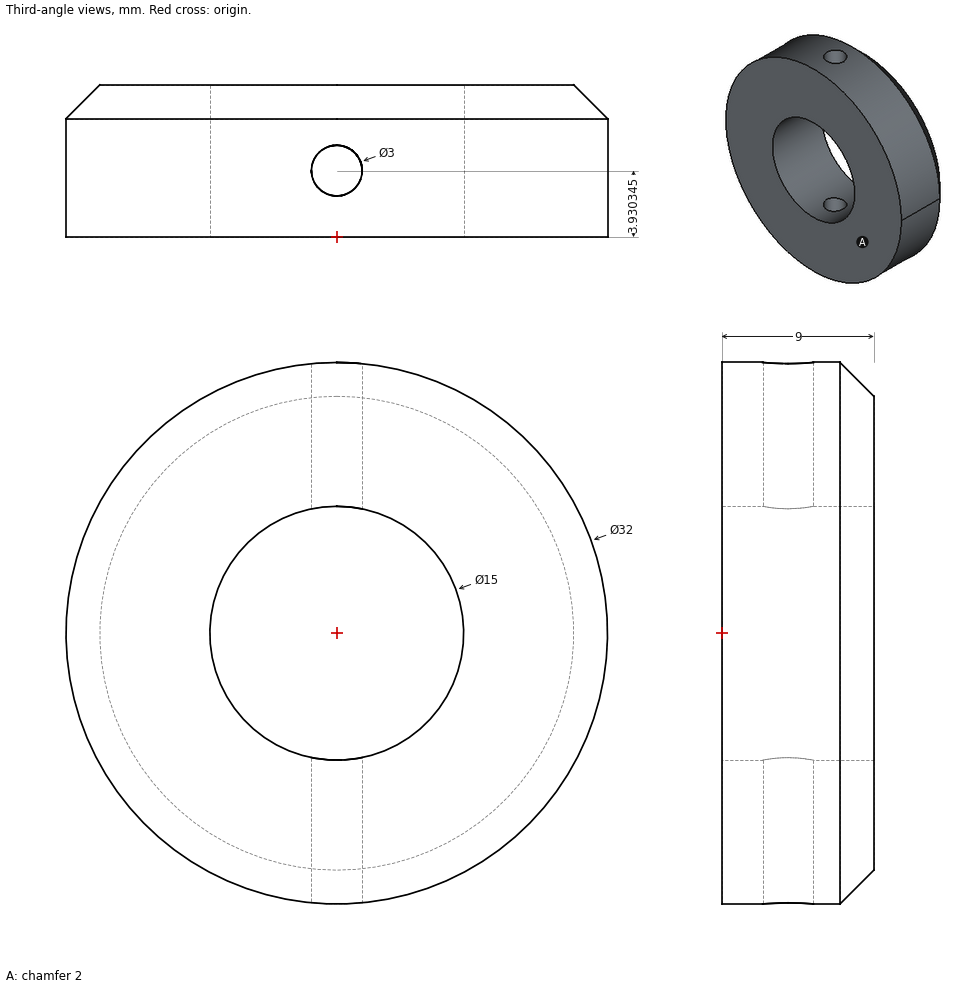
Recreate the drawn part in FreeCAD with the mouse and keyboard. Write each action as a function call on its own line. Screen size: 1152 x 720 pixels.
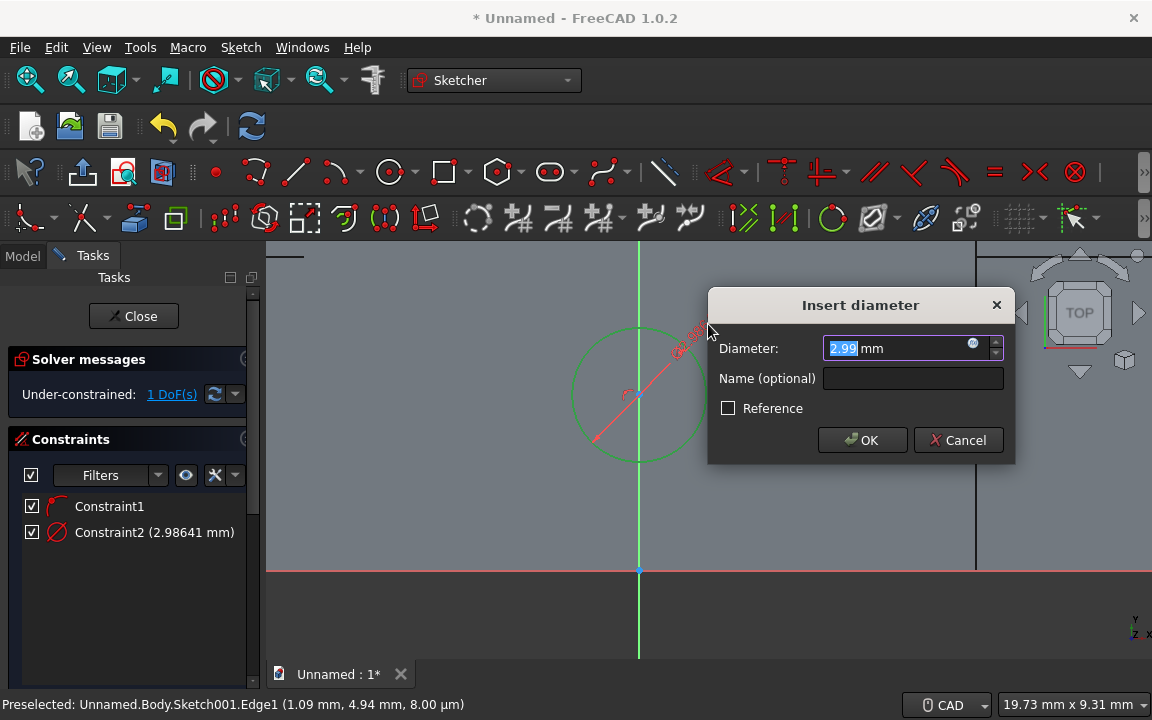
text(3)
key(Return)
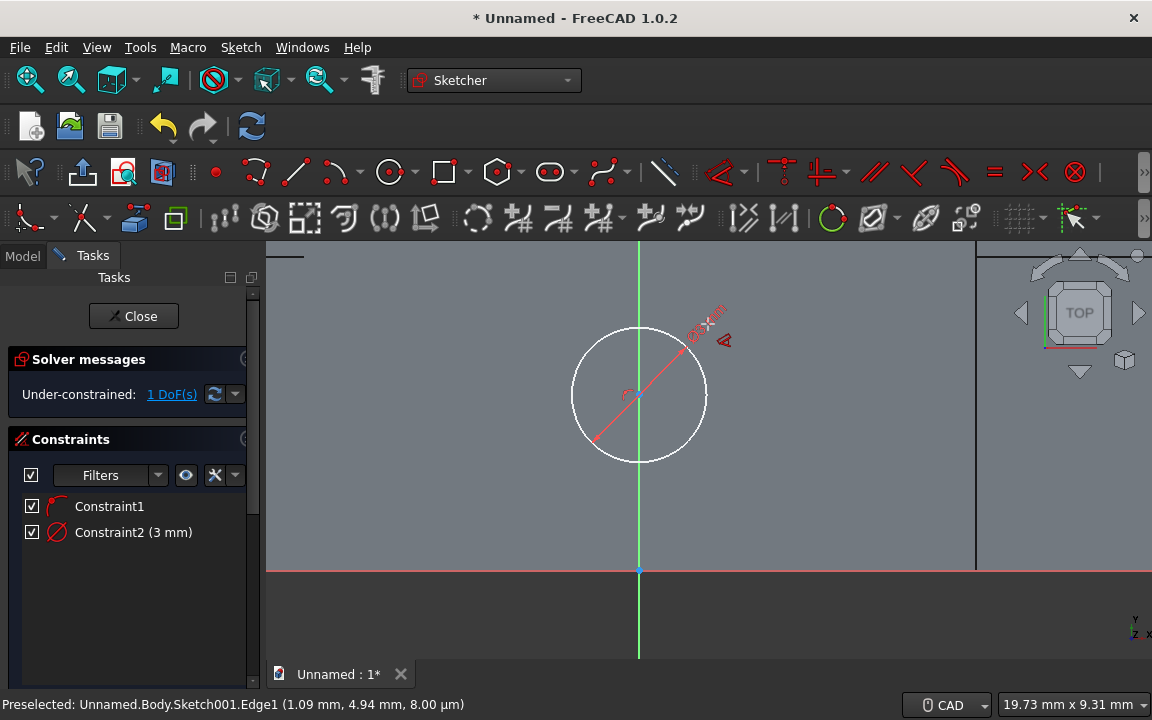
click(639, 395)
click(673, 483)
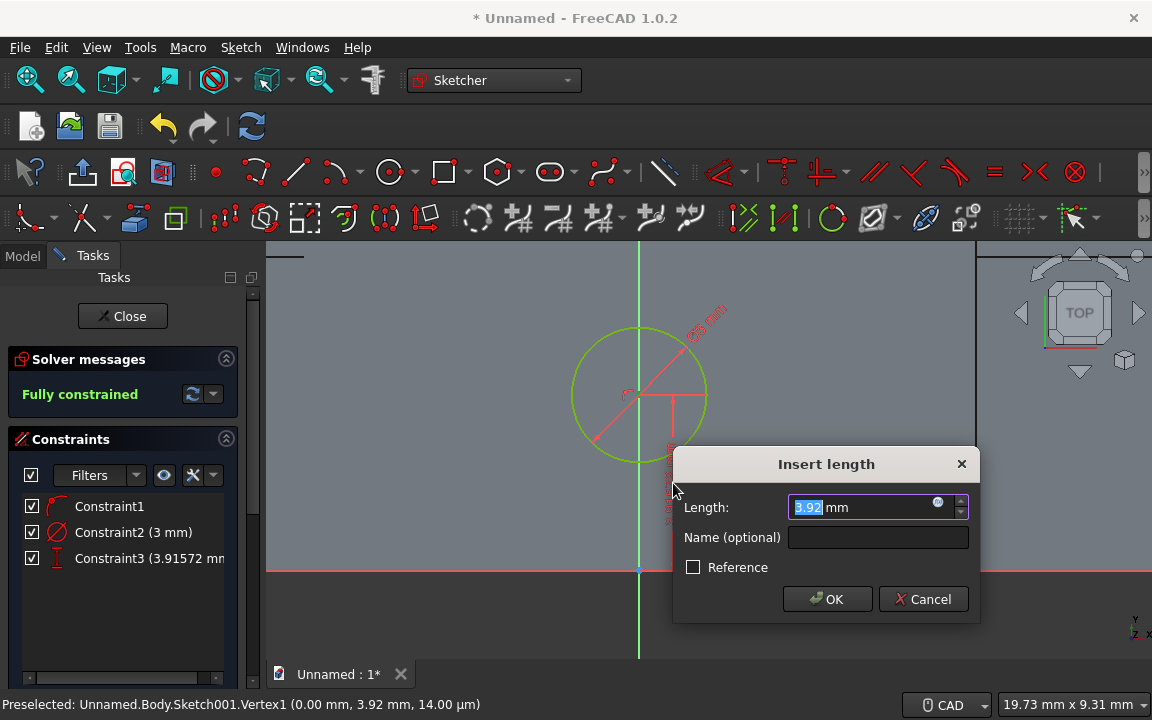
text(3.930345)
key(Return)
key(Escape)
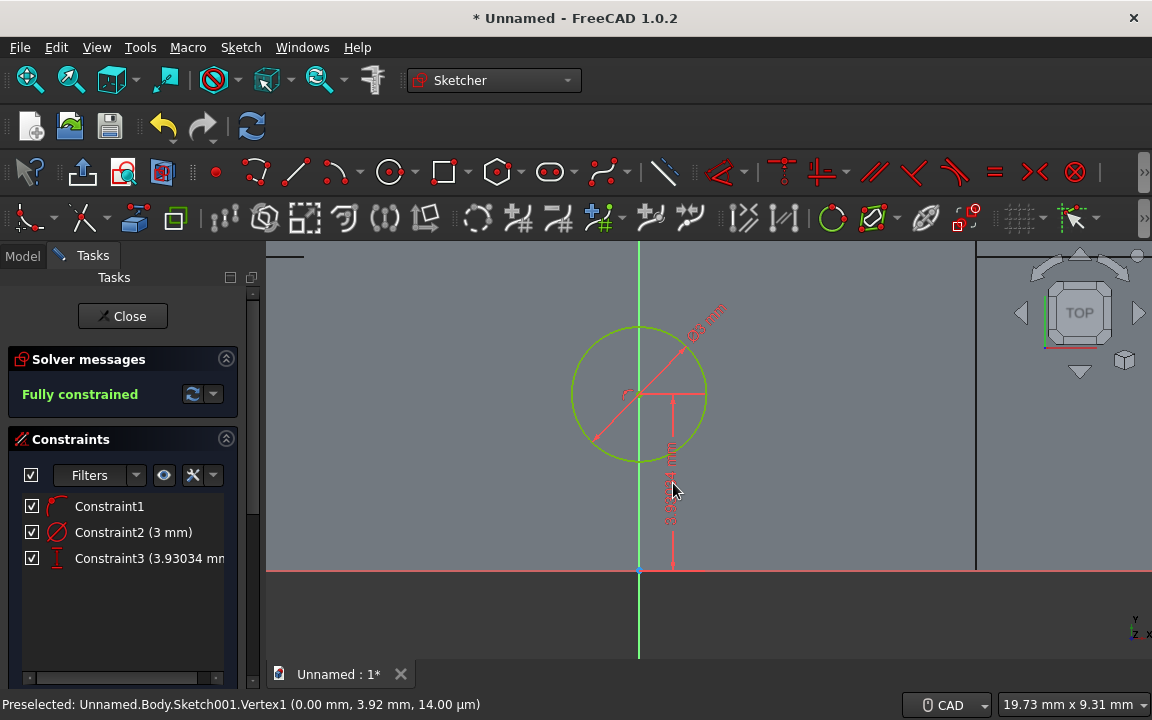
click(123, 316)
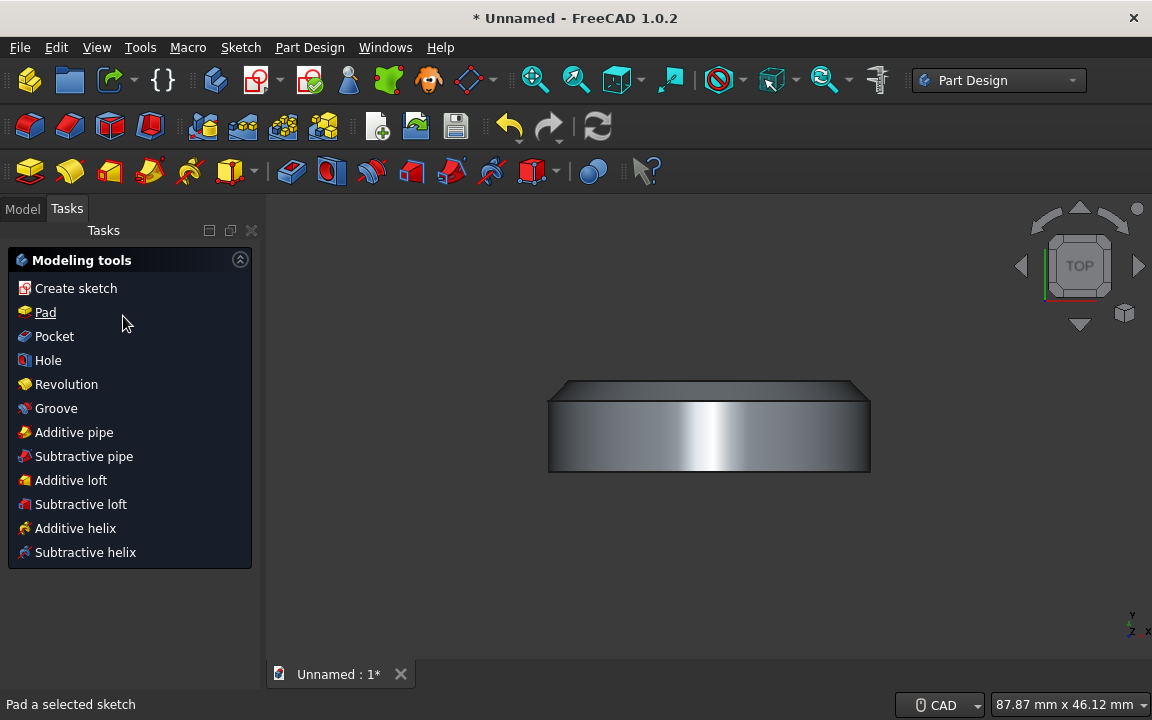
click(292, 172)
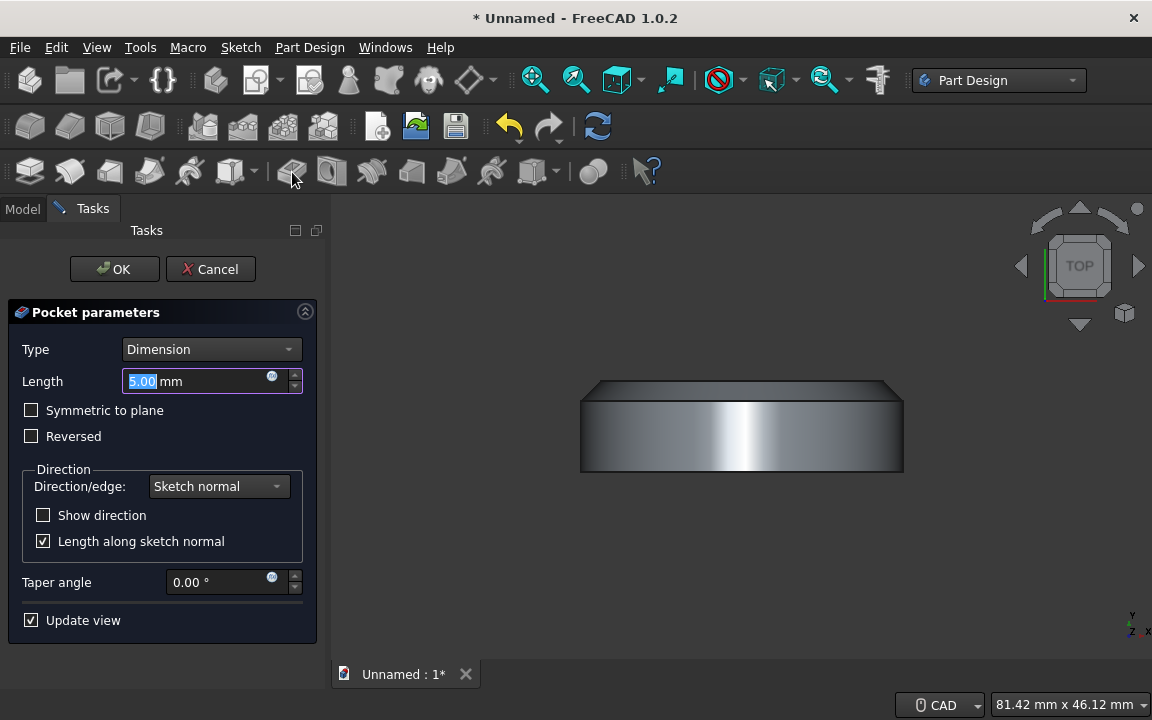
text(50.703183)
key(Tab)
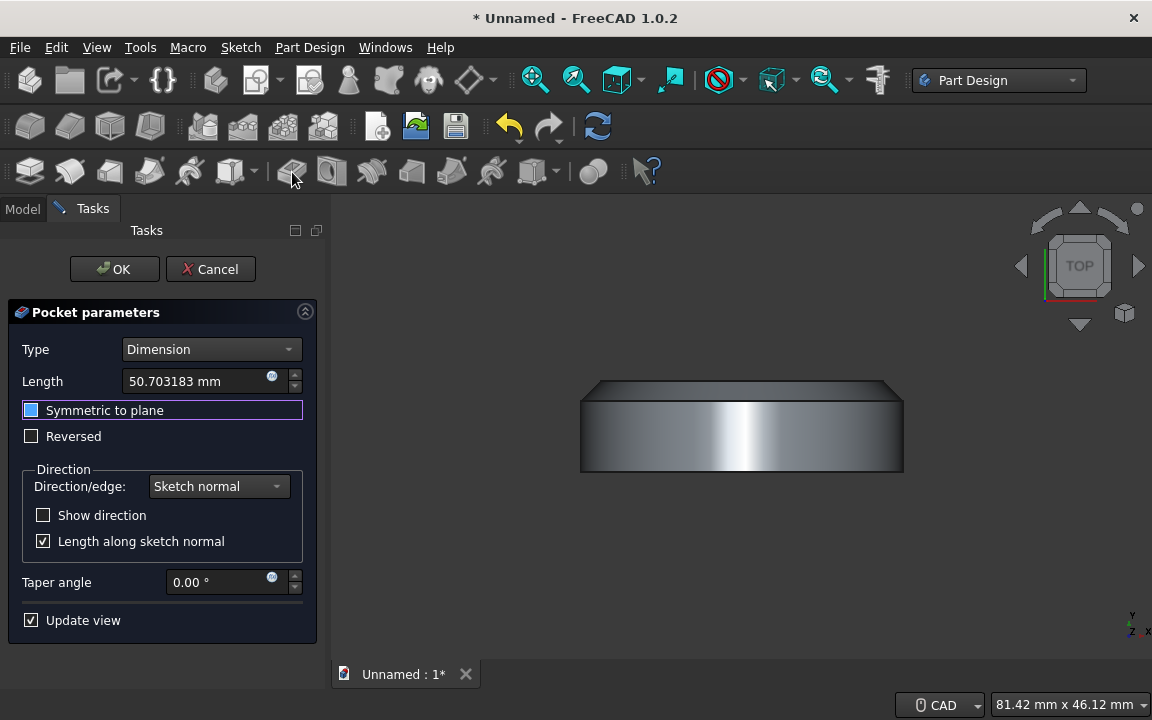
click(30, 410)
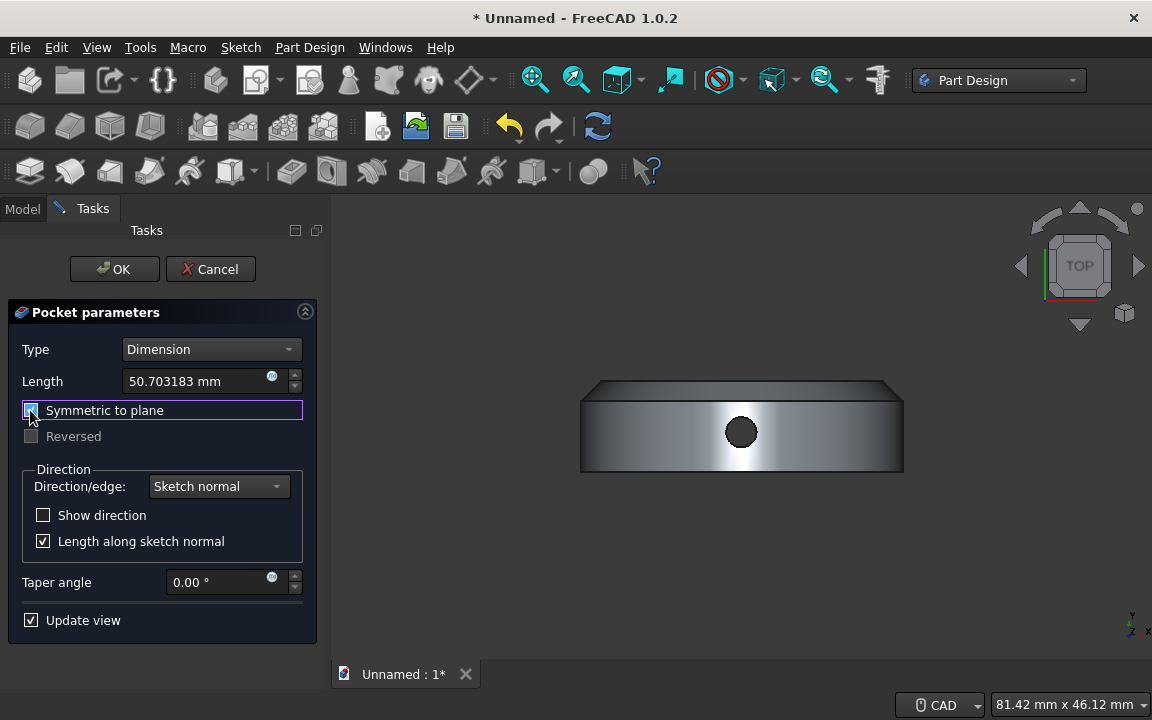
click(115, 269)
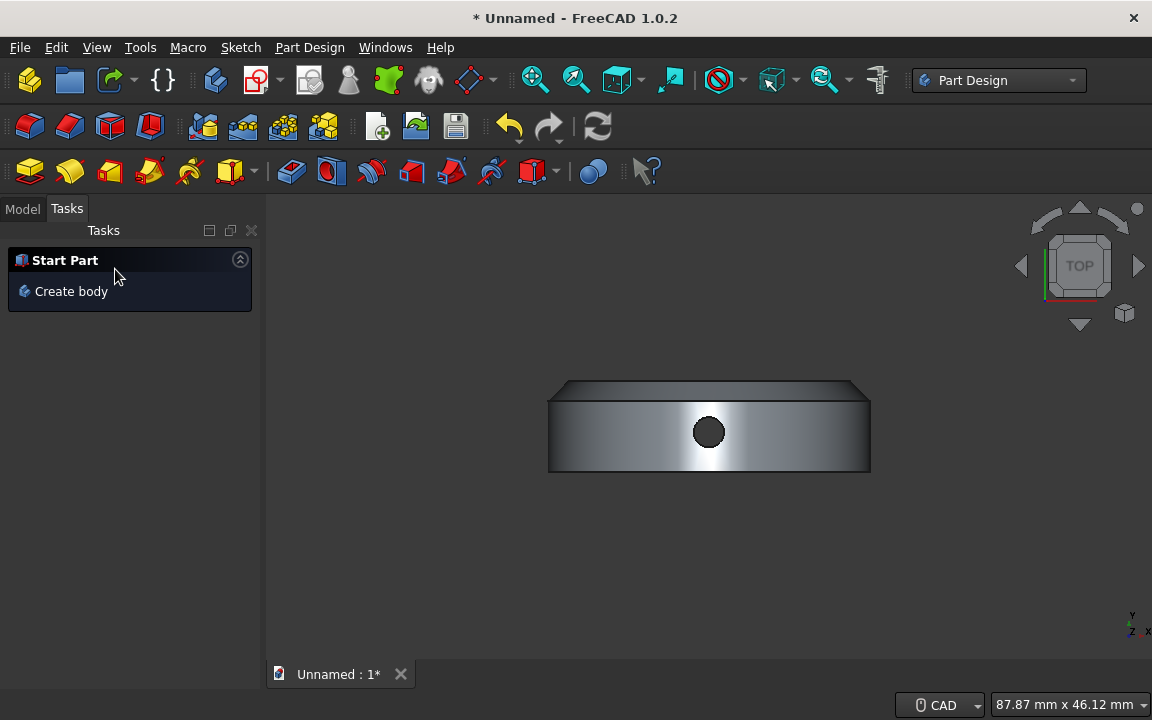
key(0)